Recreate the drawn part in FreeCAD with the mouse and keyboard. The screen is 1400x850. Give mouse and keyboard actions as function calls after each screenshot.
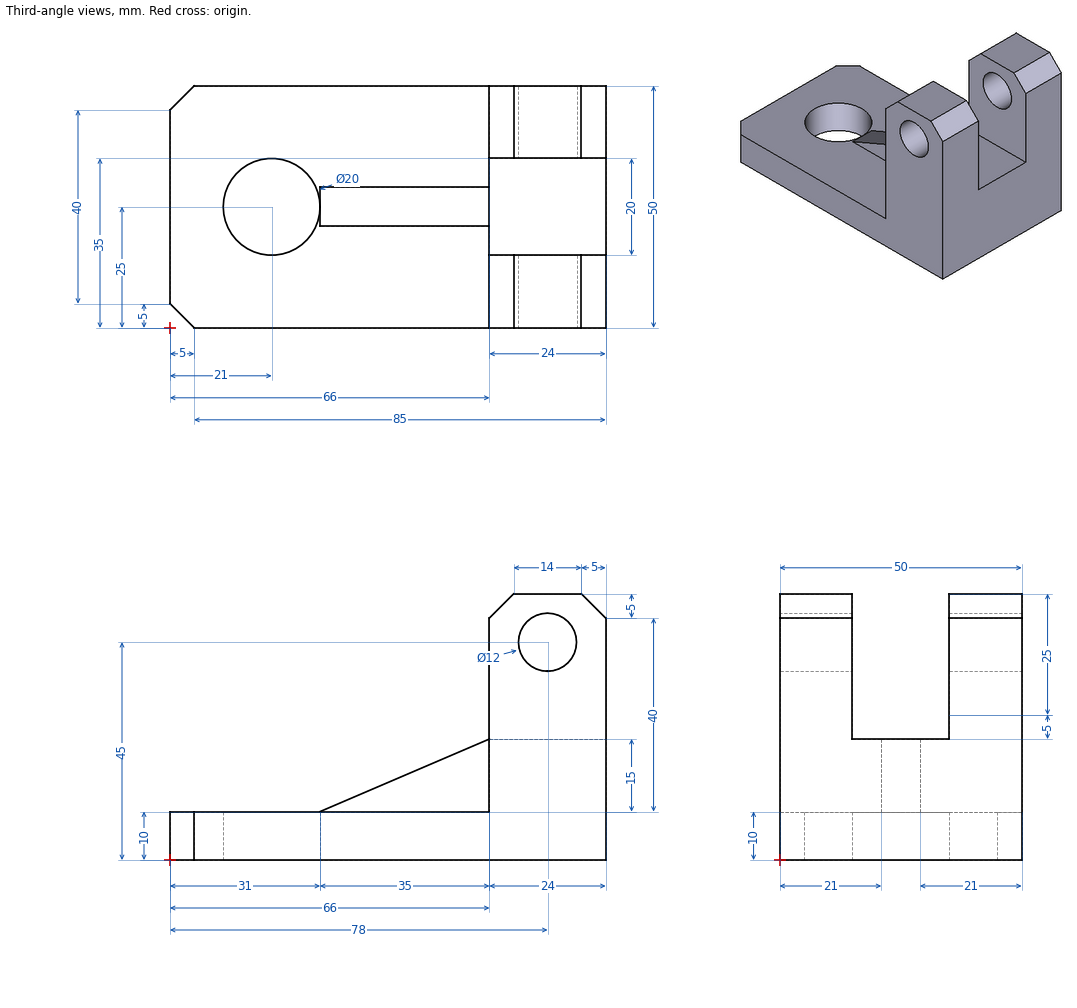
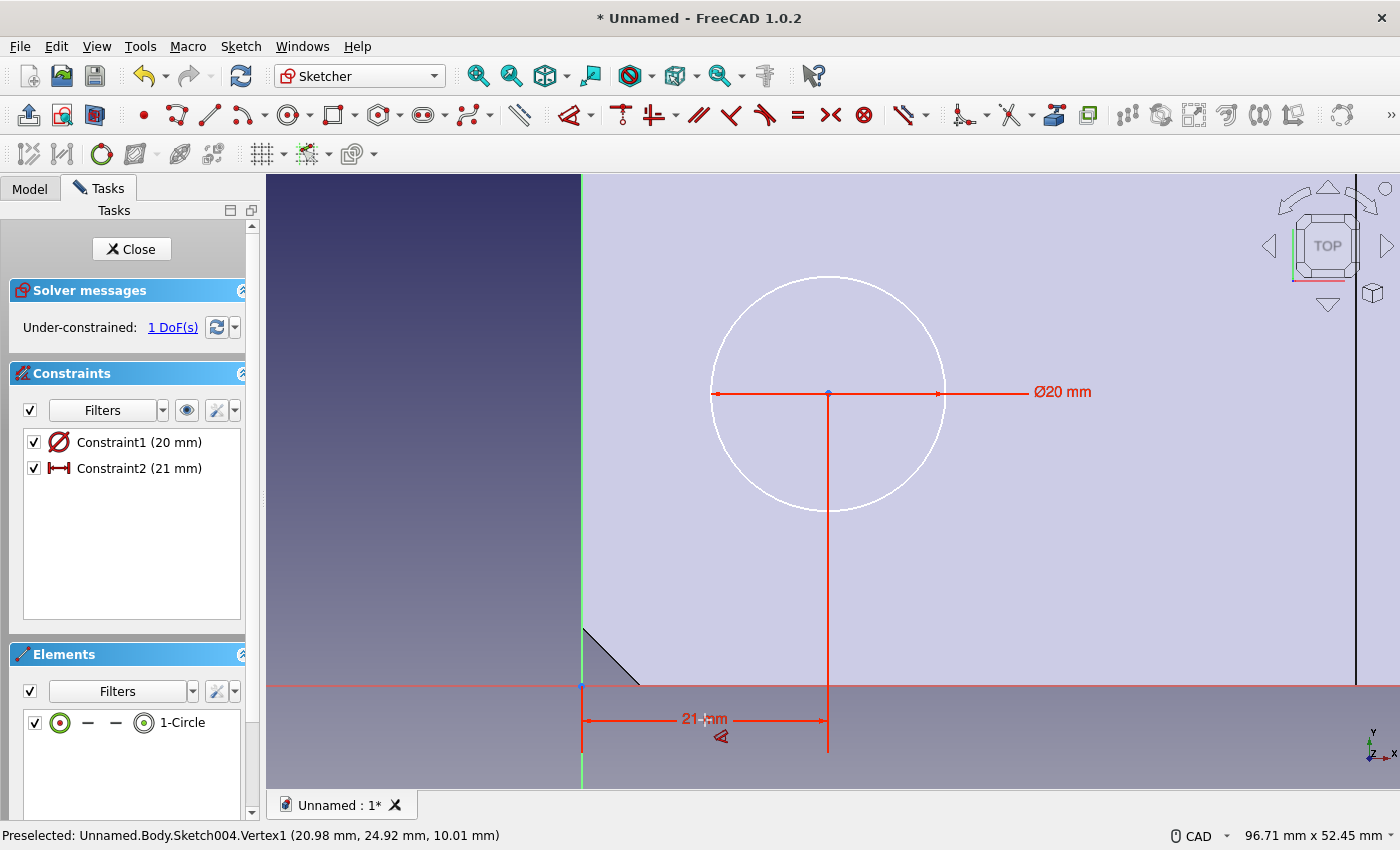
click(828, 394)
click(548, 540)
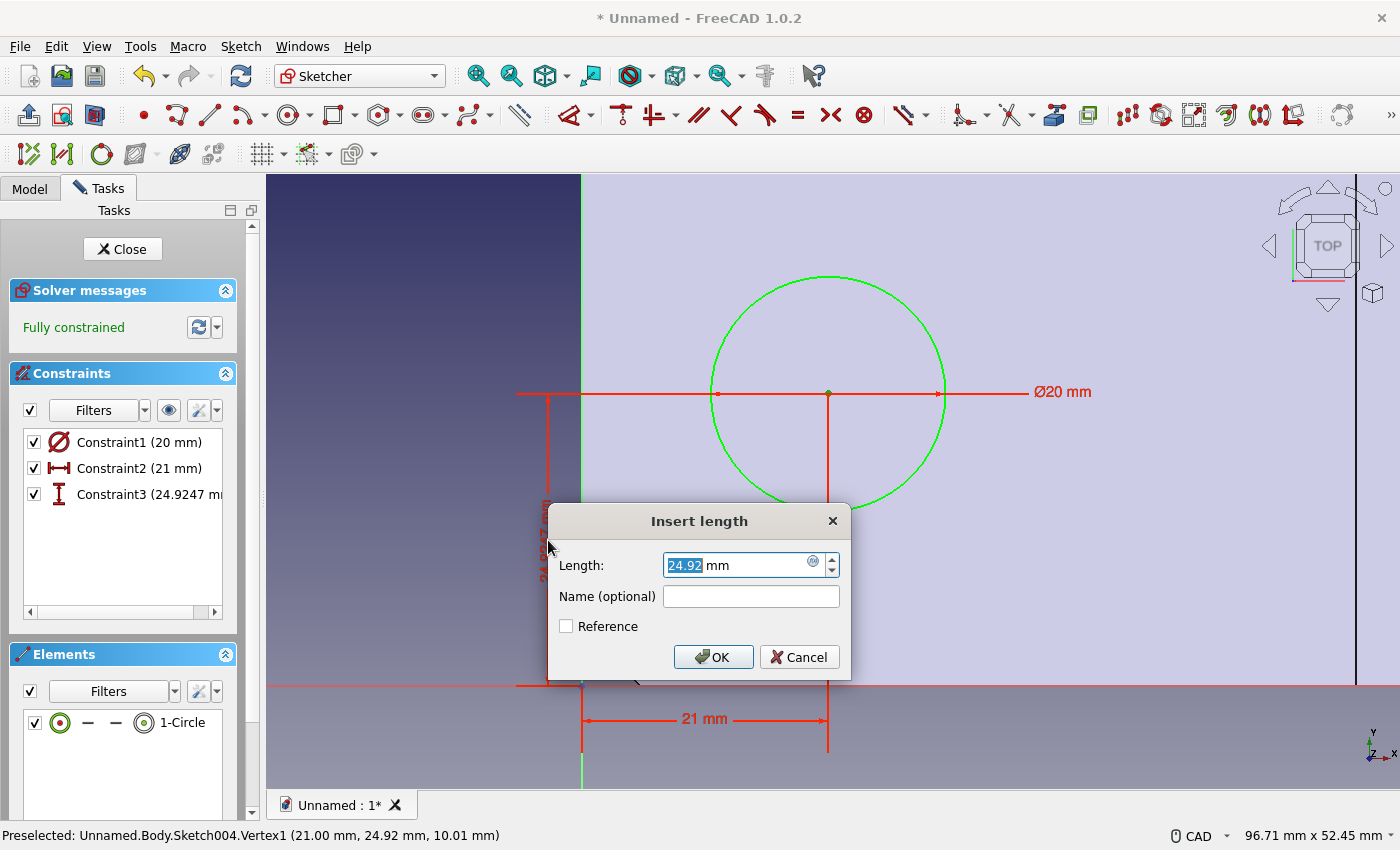
text(25)
key(Return)
key(Escape)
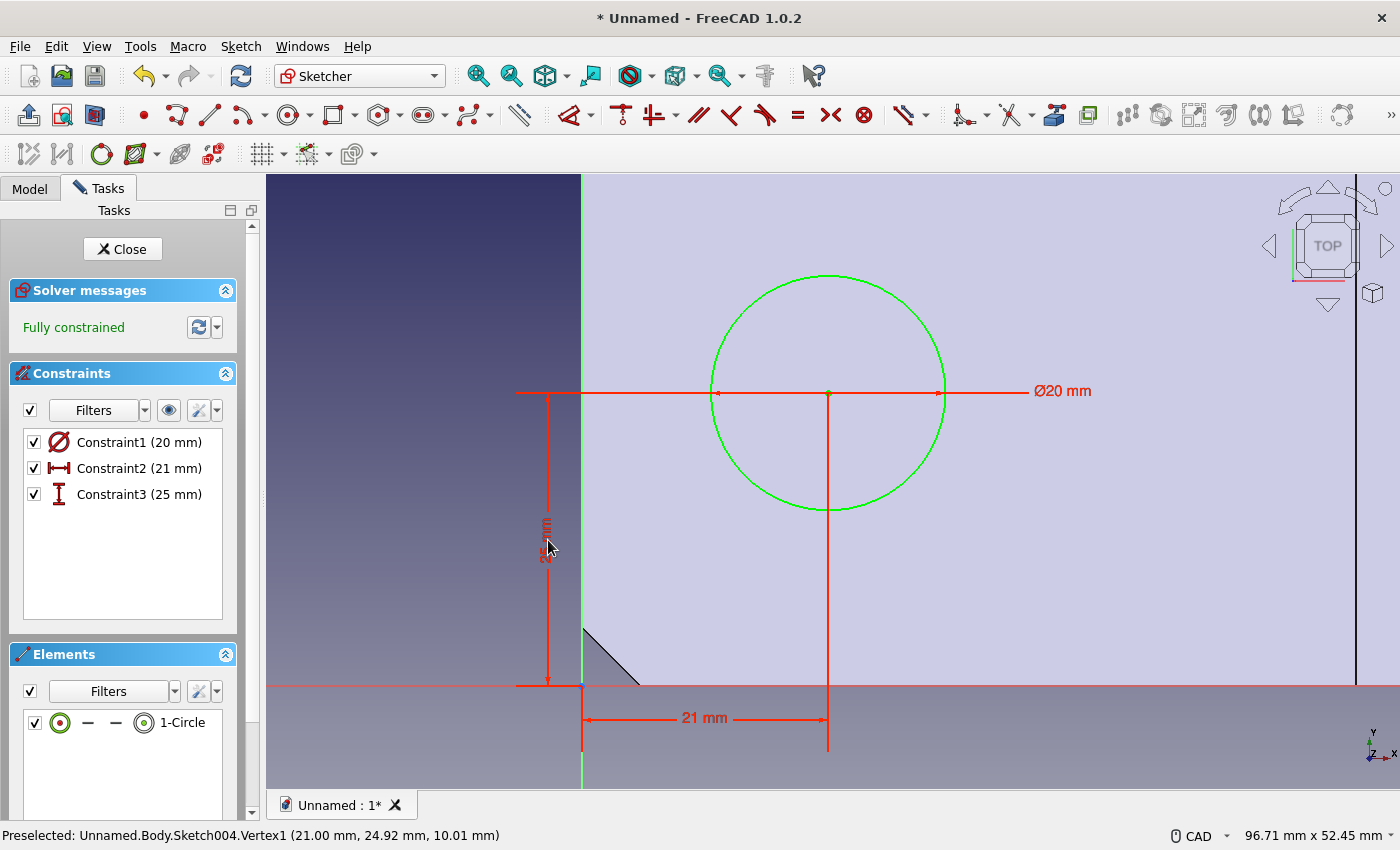
click(123, 249)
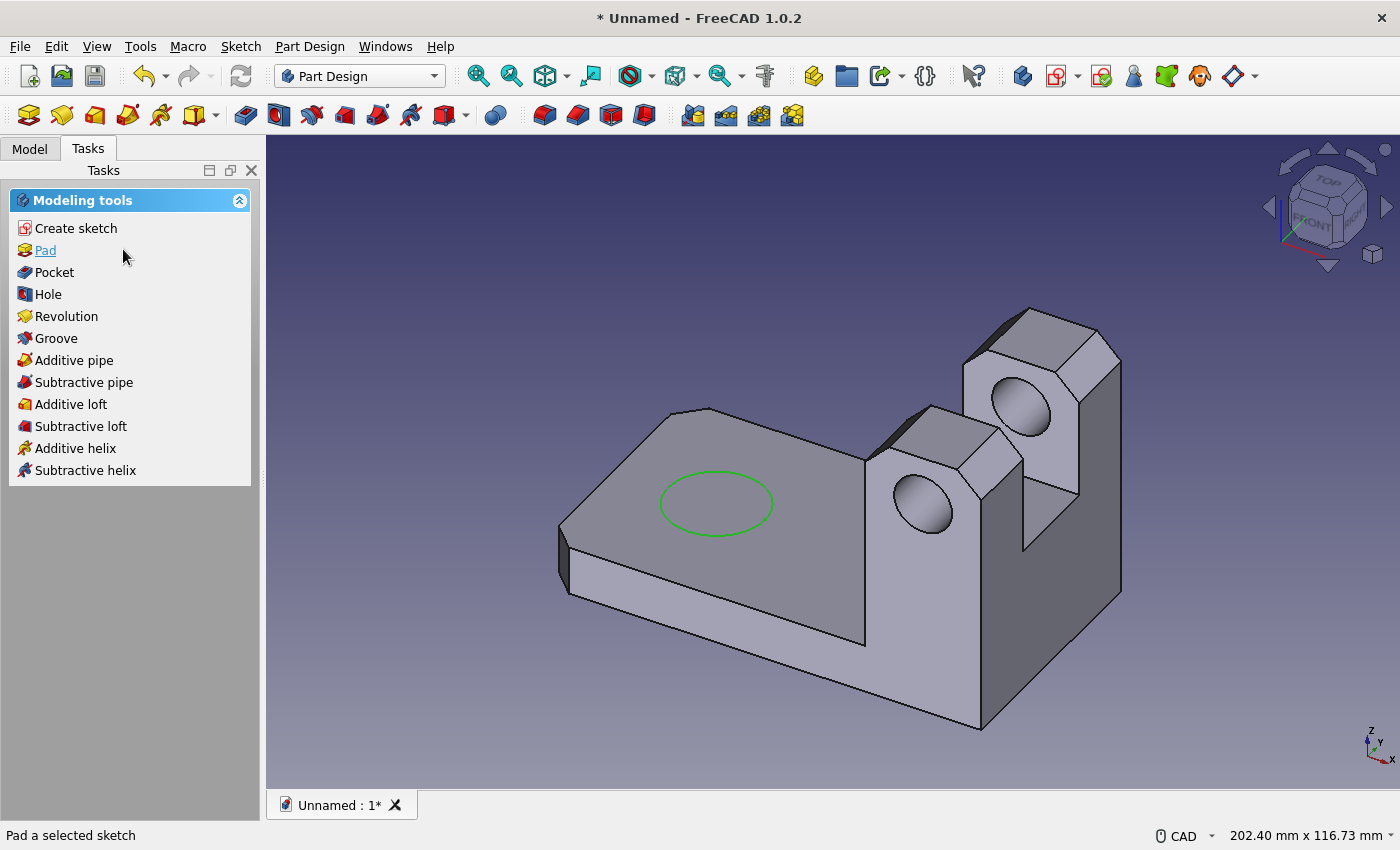
click(246, 116)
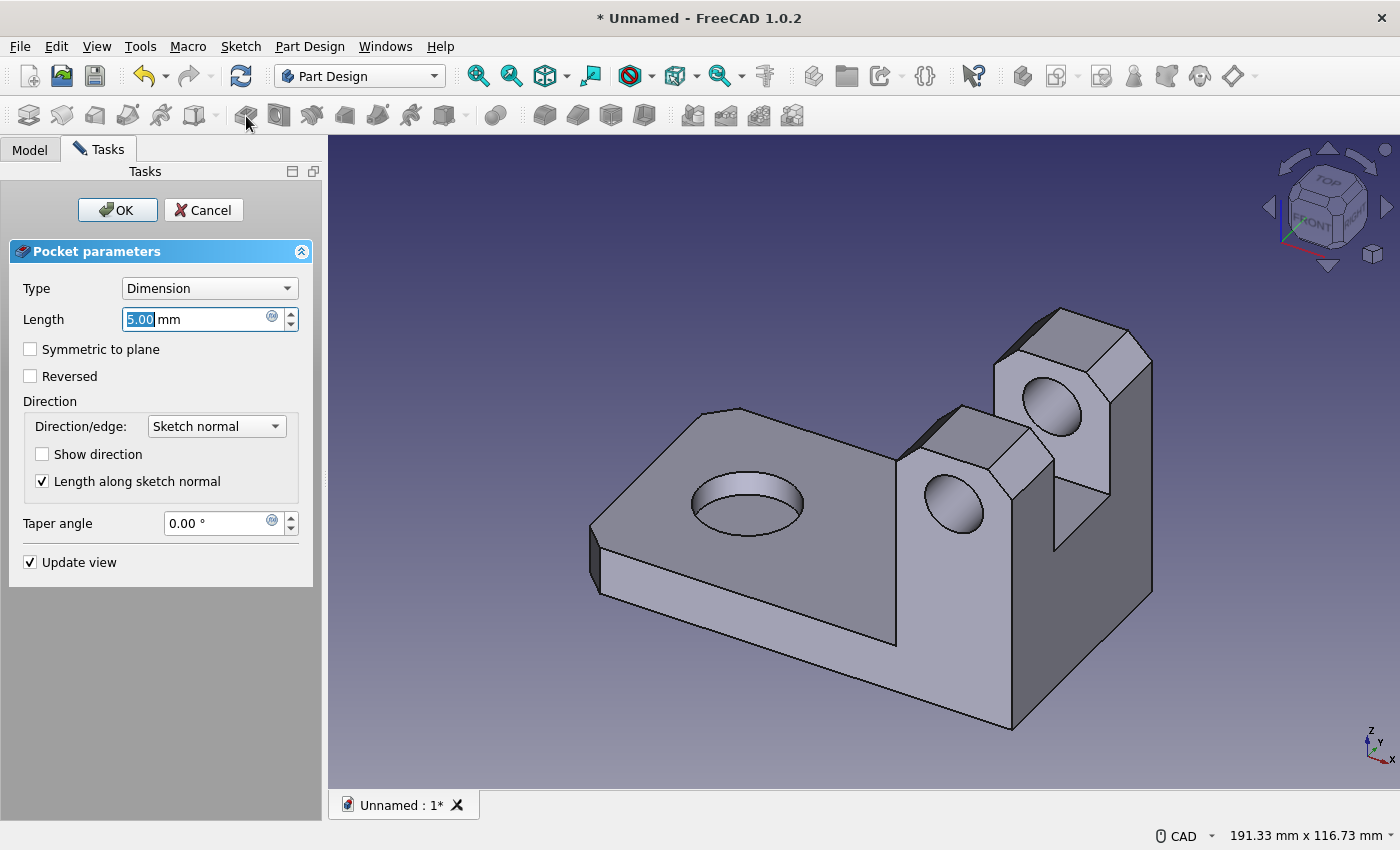
text(10)
key(Tab)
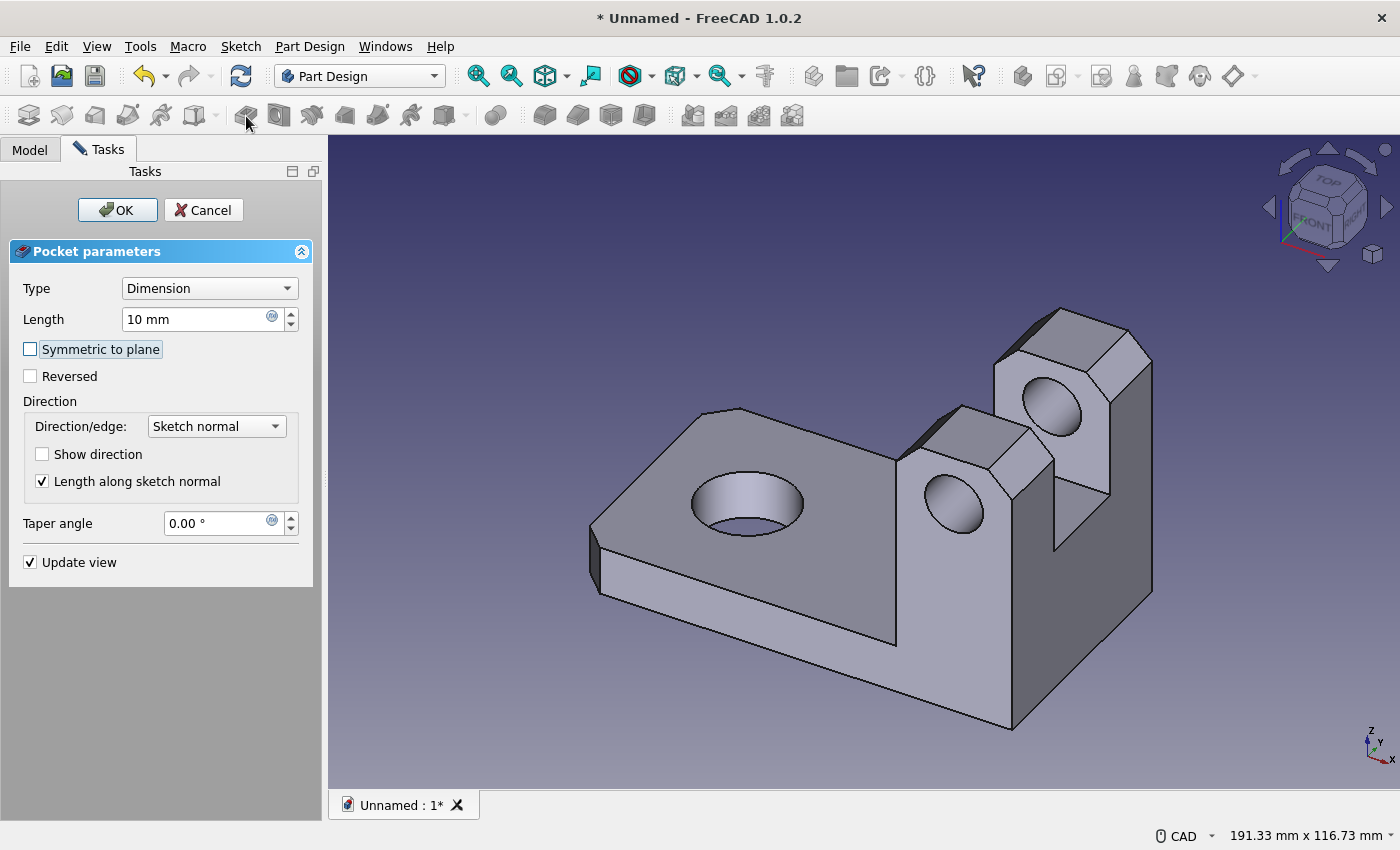
click(118, 210)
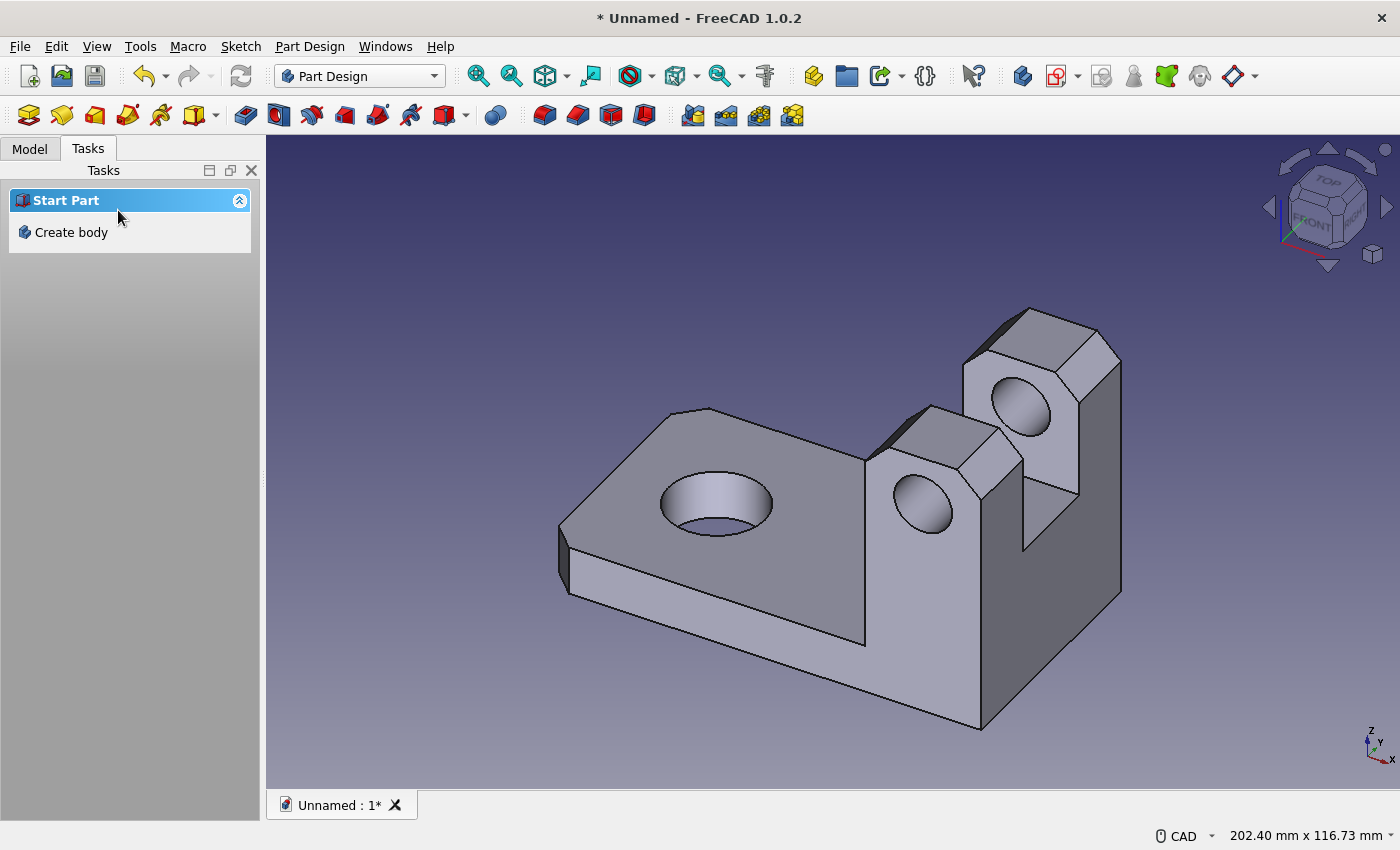
click(1056, 76)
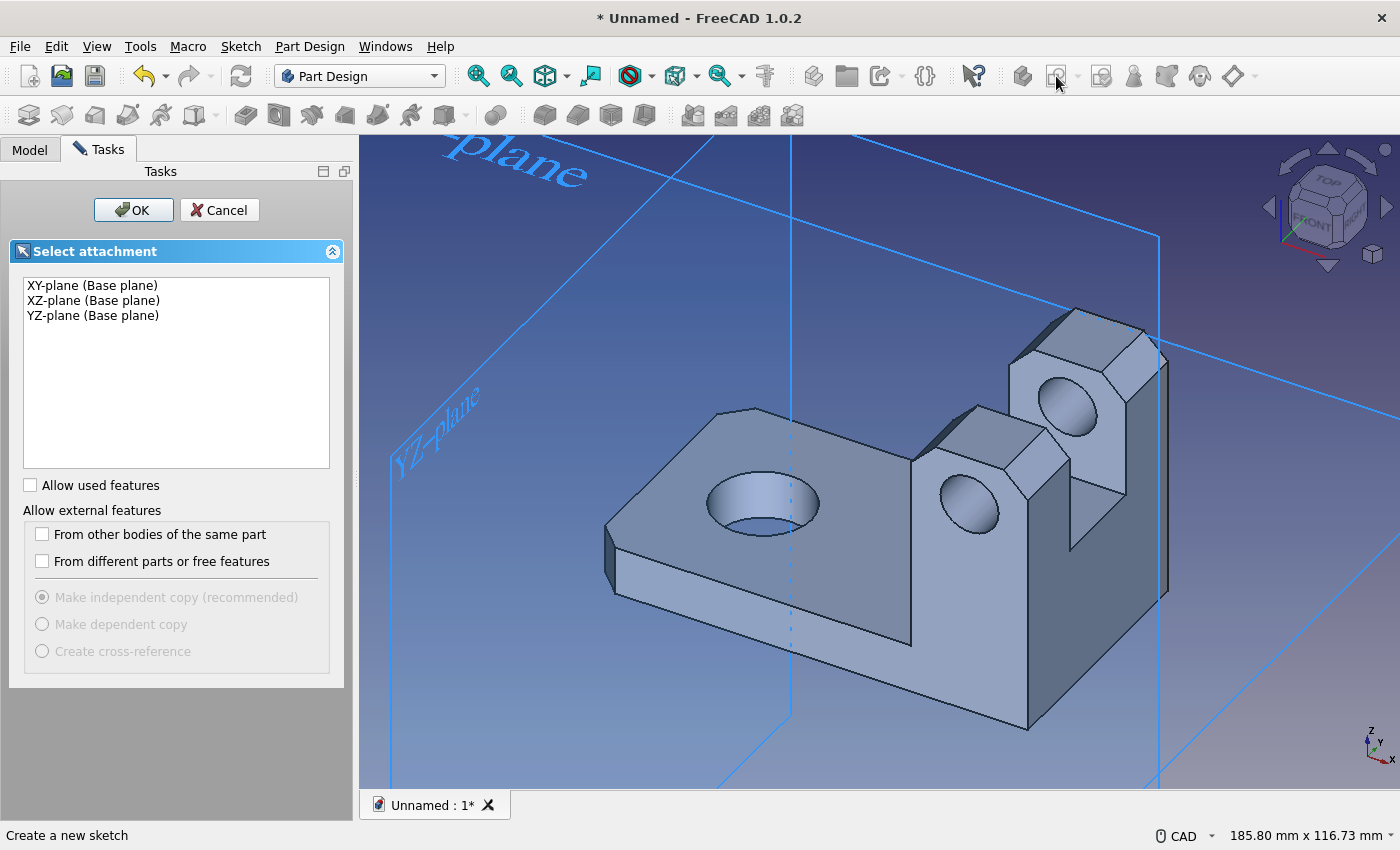
click(84, 300)